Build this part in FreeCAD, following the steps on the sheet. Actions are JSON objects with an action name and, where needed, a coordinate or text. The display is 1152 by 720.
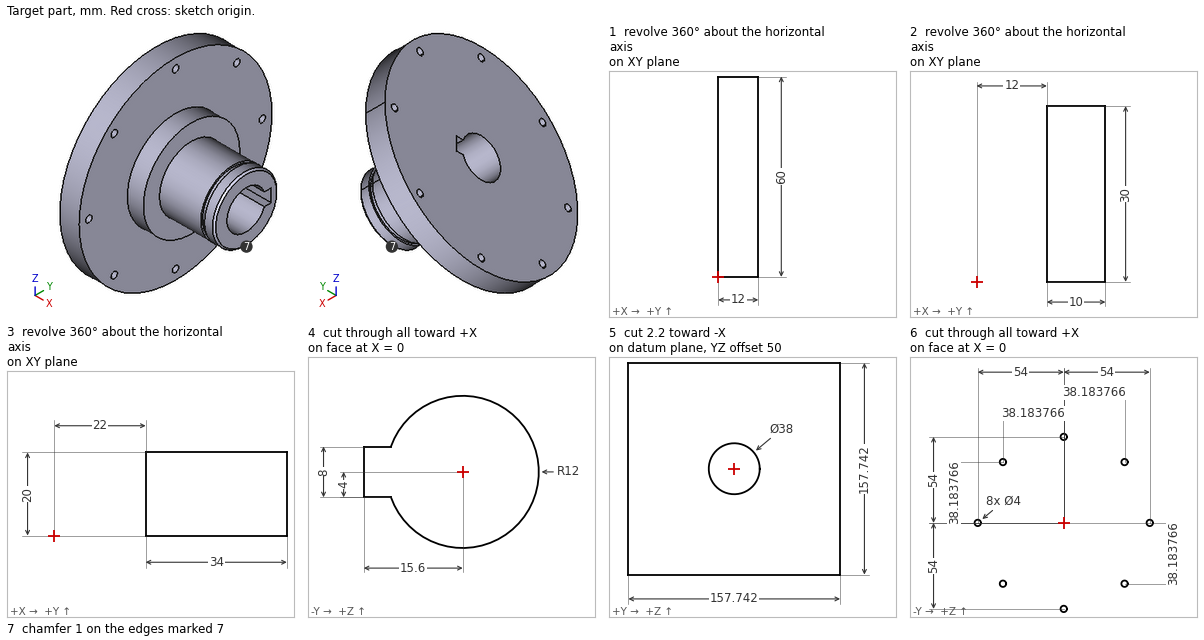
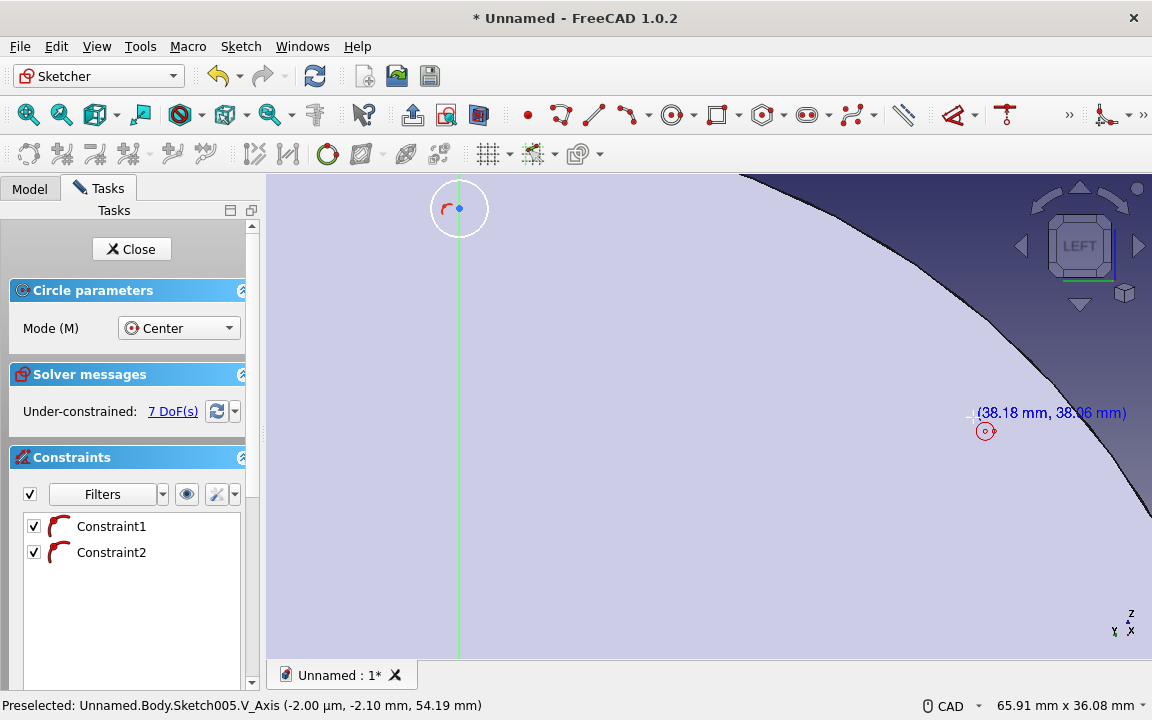
{"action": "scroll", "coordinate": [686, 287], "scroll_direction": "down", "scroll_amount": 8}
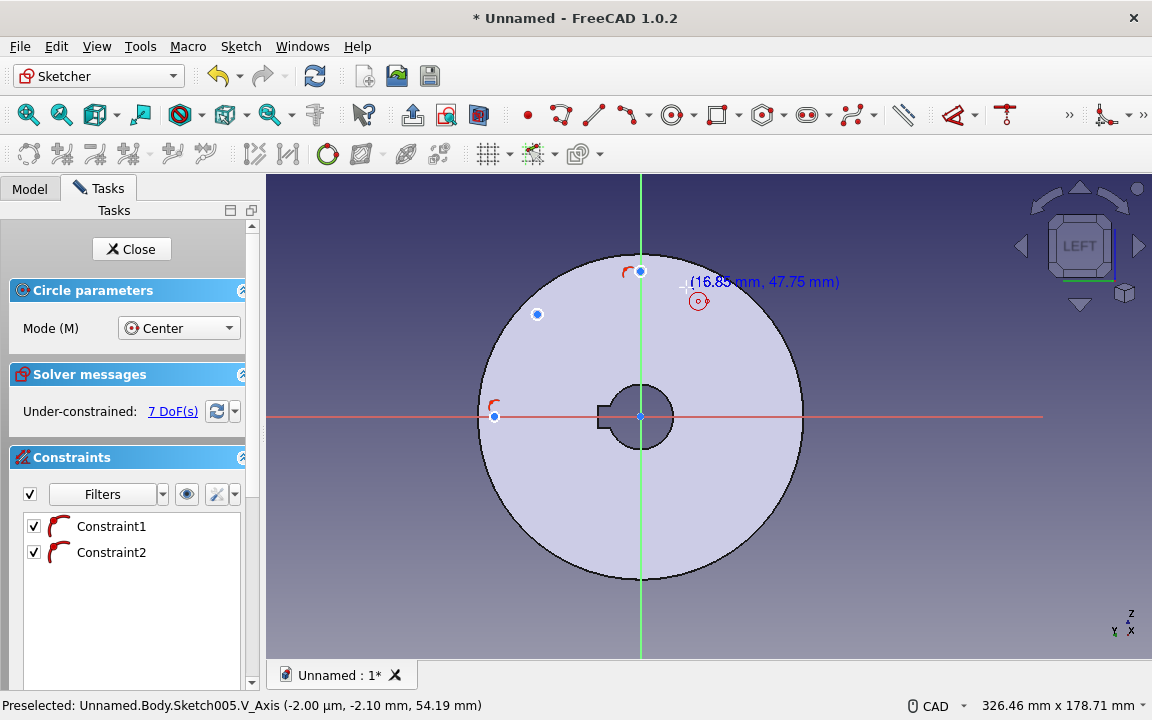
{"action": "left_click", "coordinate": [744, 313]}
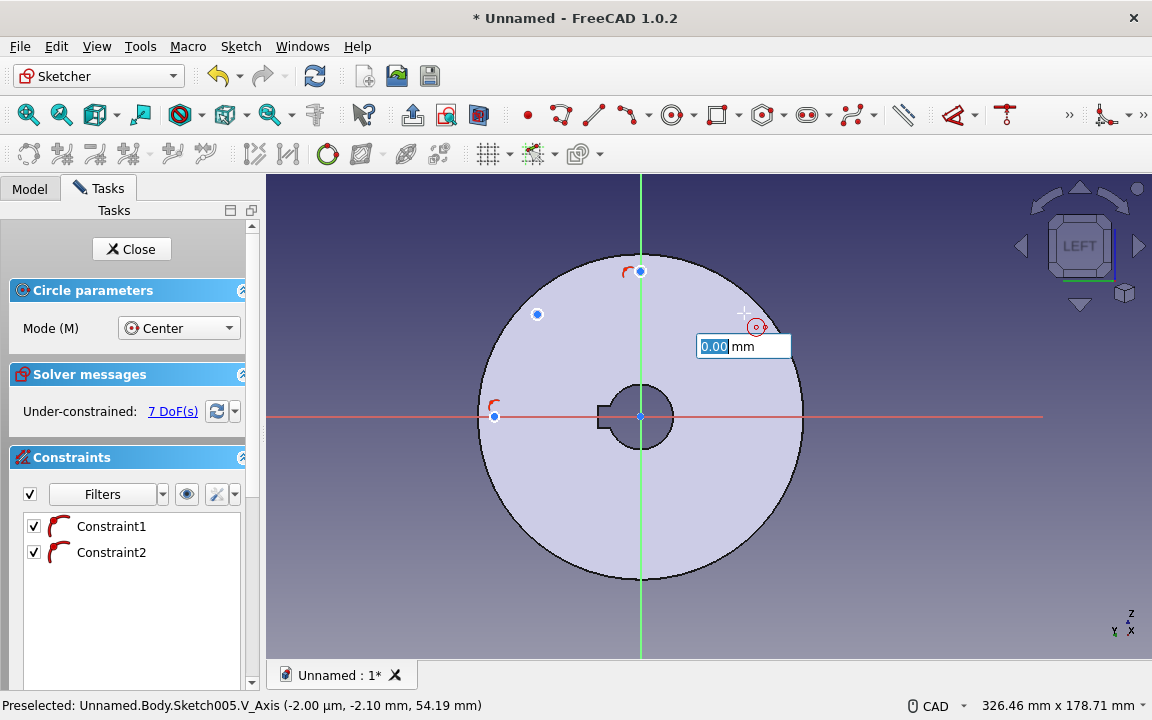
{"action": "scroll", "coordinate": [748, 310], "scroll_direction": "up", "scroll_amount": 6}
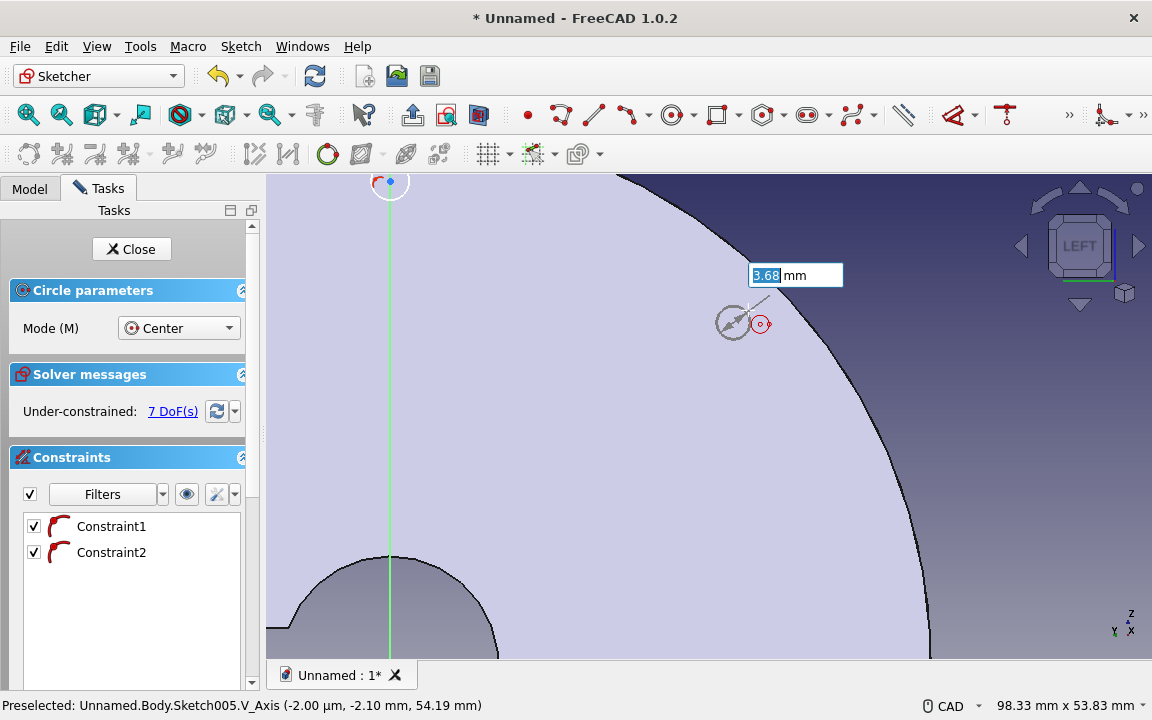
{"action": "left_click", "coordinate": [747, 308]}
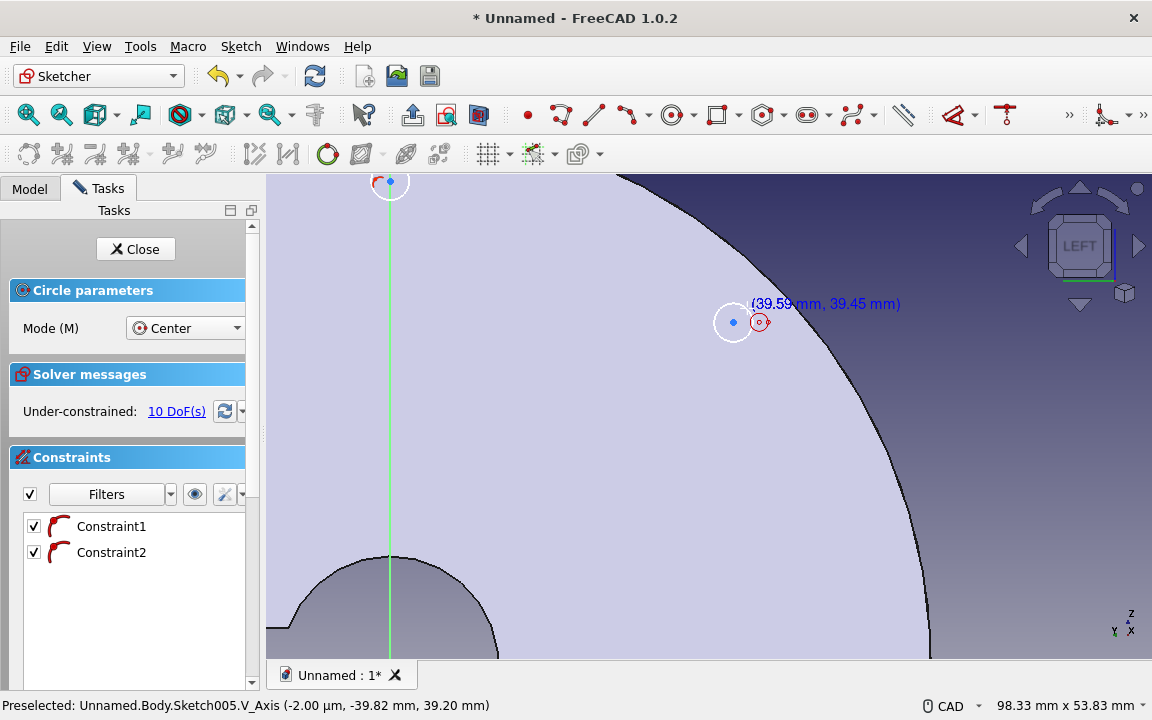
{"action": "scroll", "coordinate": [748, 310], "scroll_direction": "down", "scroll_amount": 6}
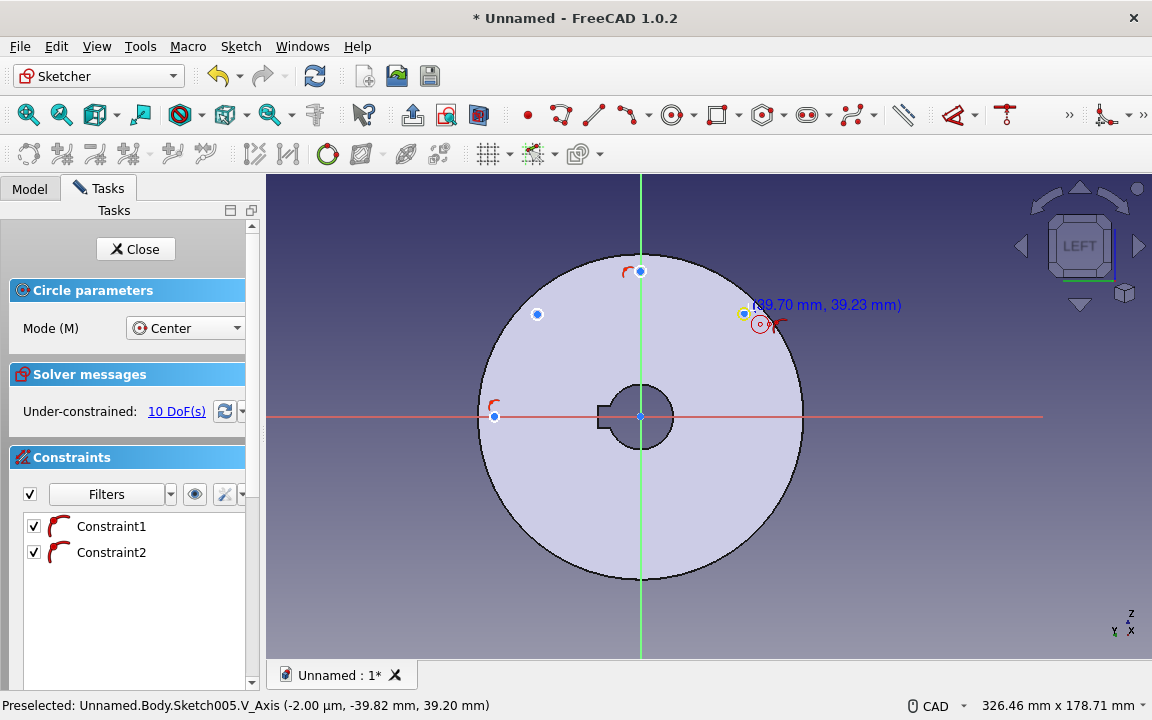
{"action": "scroll", "coordinate": [787, 417], "scroll_direction": "up", "scroll_amount": 8}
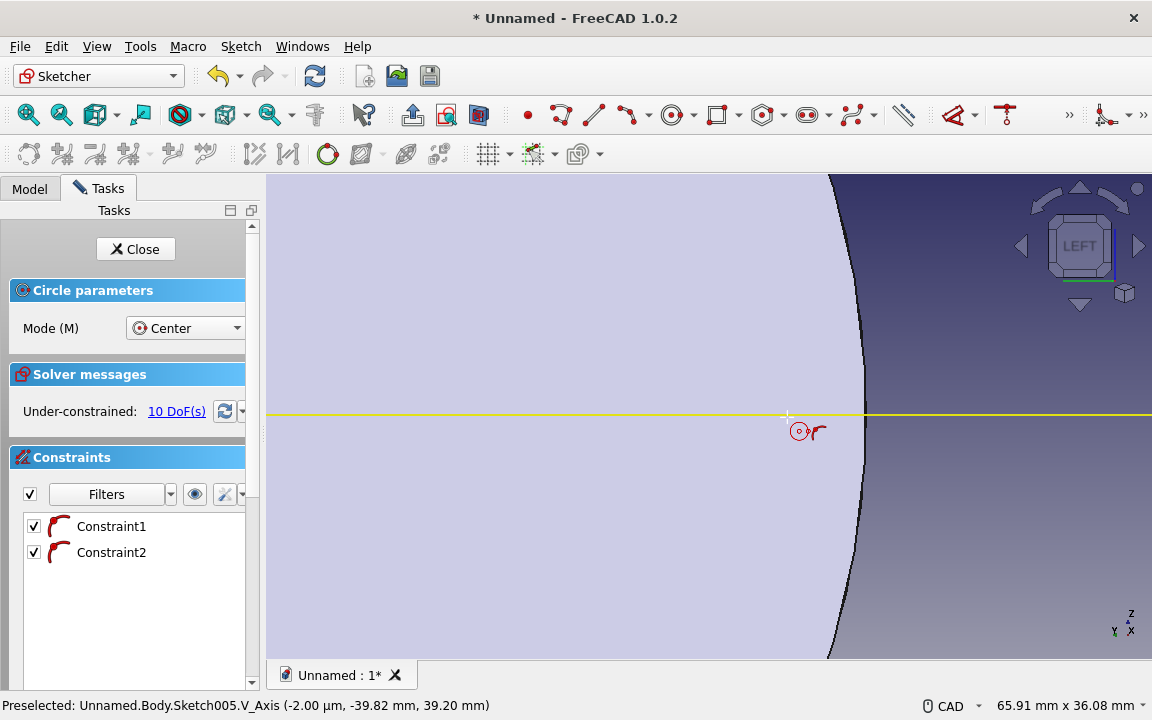
{"action": "scroll", "coordinate": [787, 417], "scroll_direction": "down", "scroll_amount": 8}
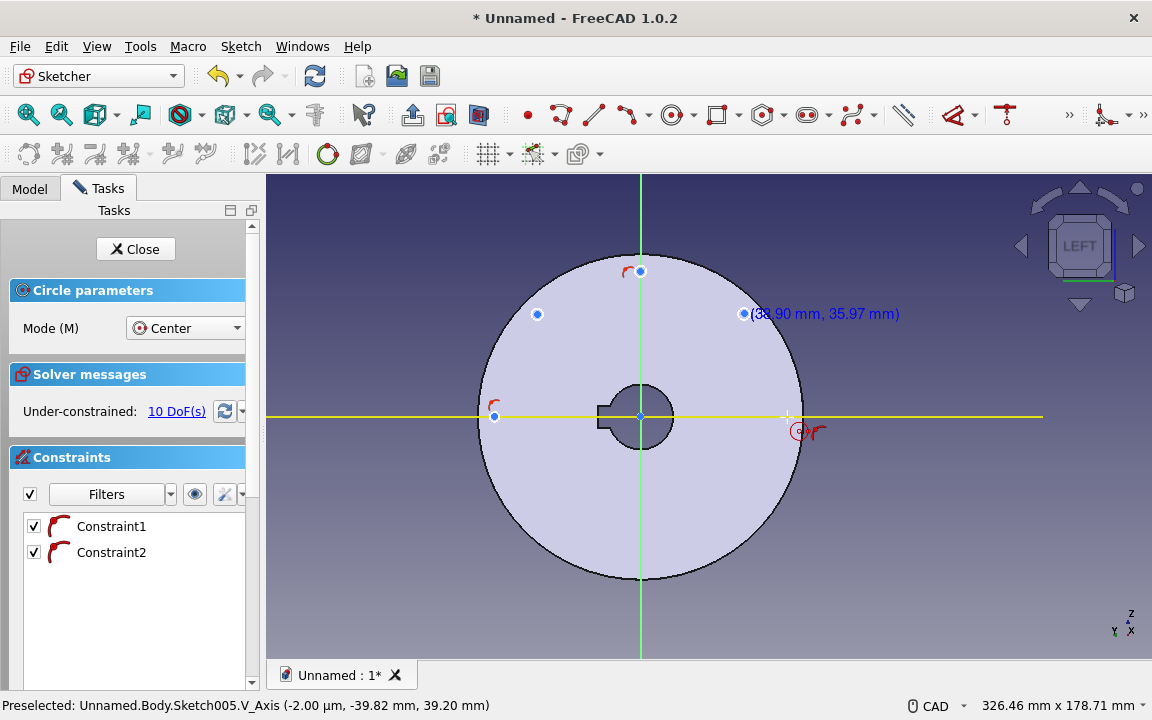
{"action": "left_click", "coordinate": [787, 417]}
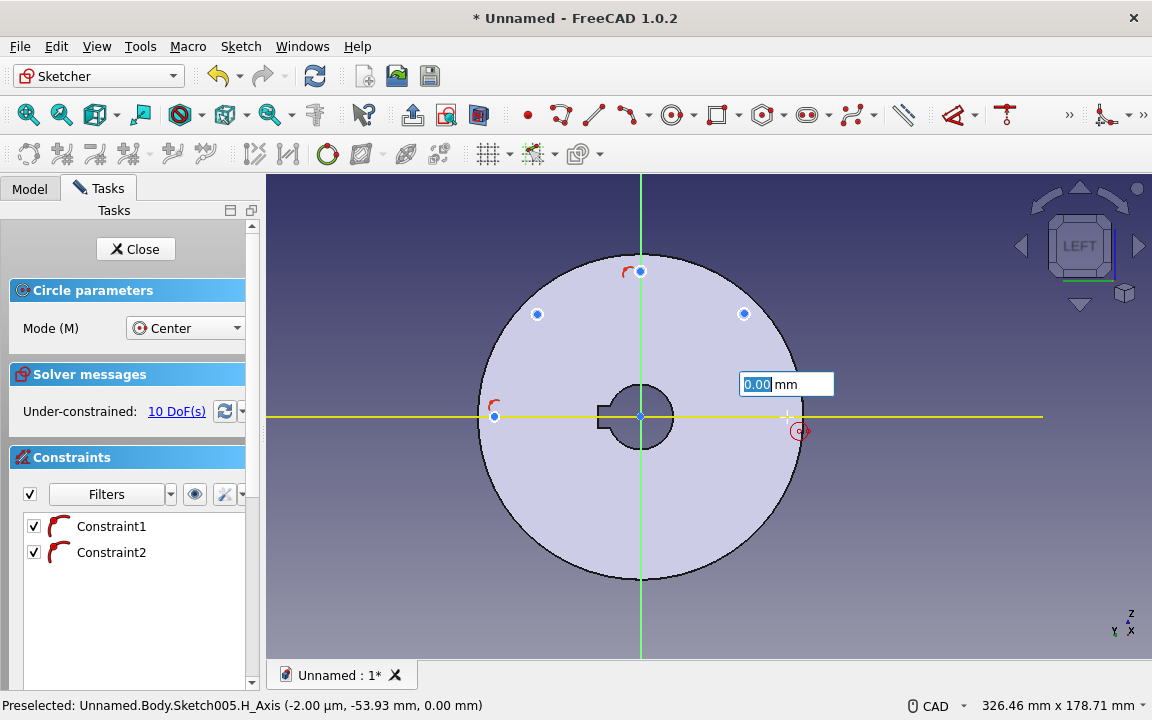
{"action": "scroll", "coordinate": [785, 422], "scroll_direction": "up", "scroll_amount": 6}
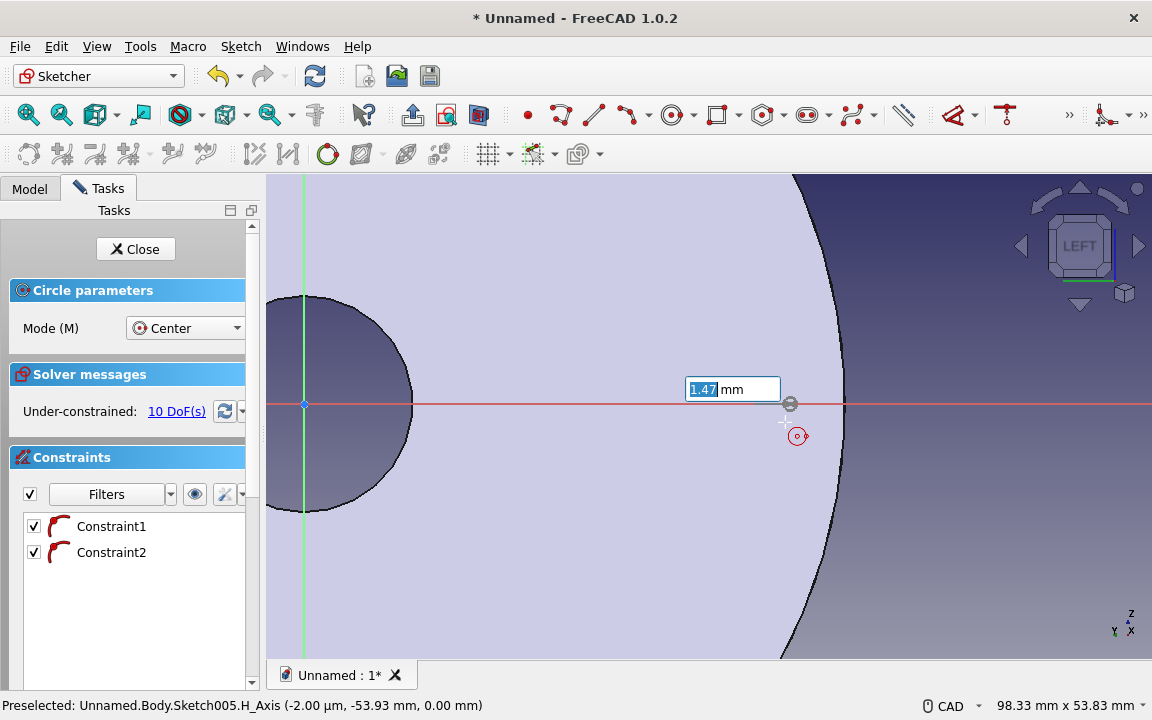
{"action": "left_click", "coordinate": [785, 421]}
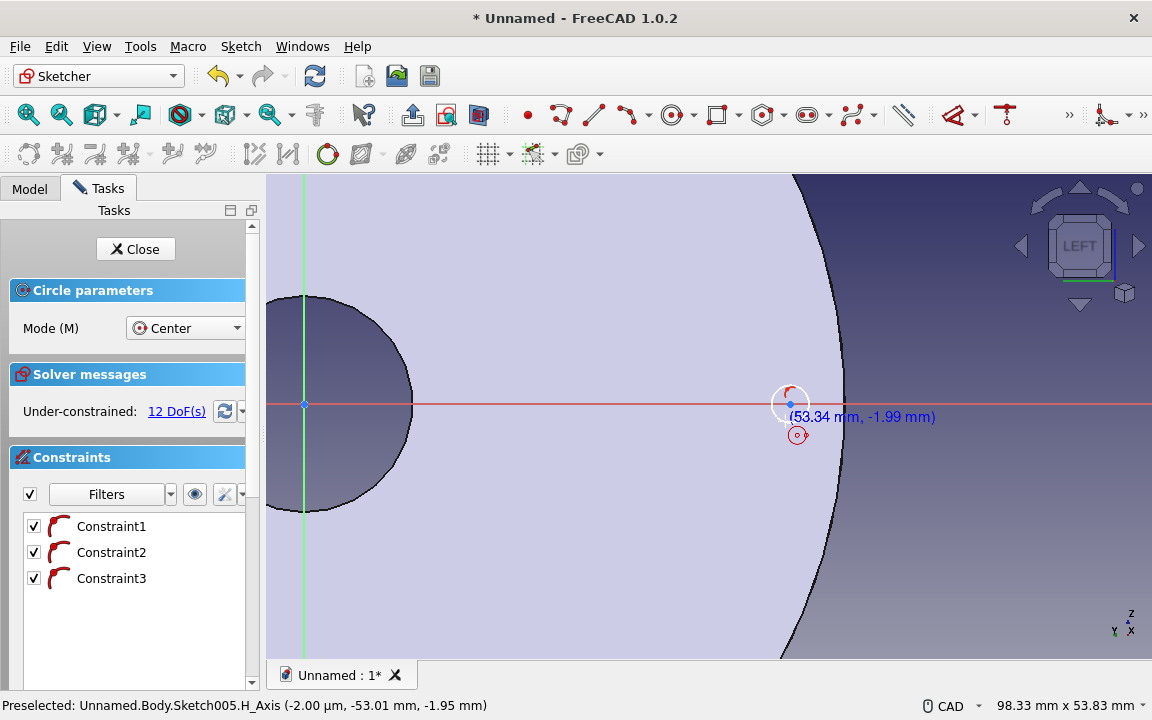
{"action": "scroll", "coordinate": [785, 422], "scroll_direction": "down", "scroll_amount": 6}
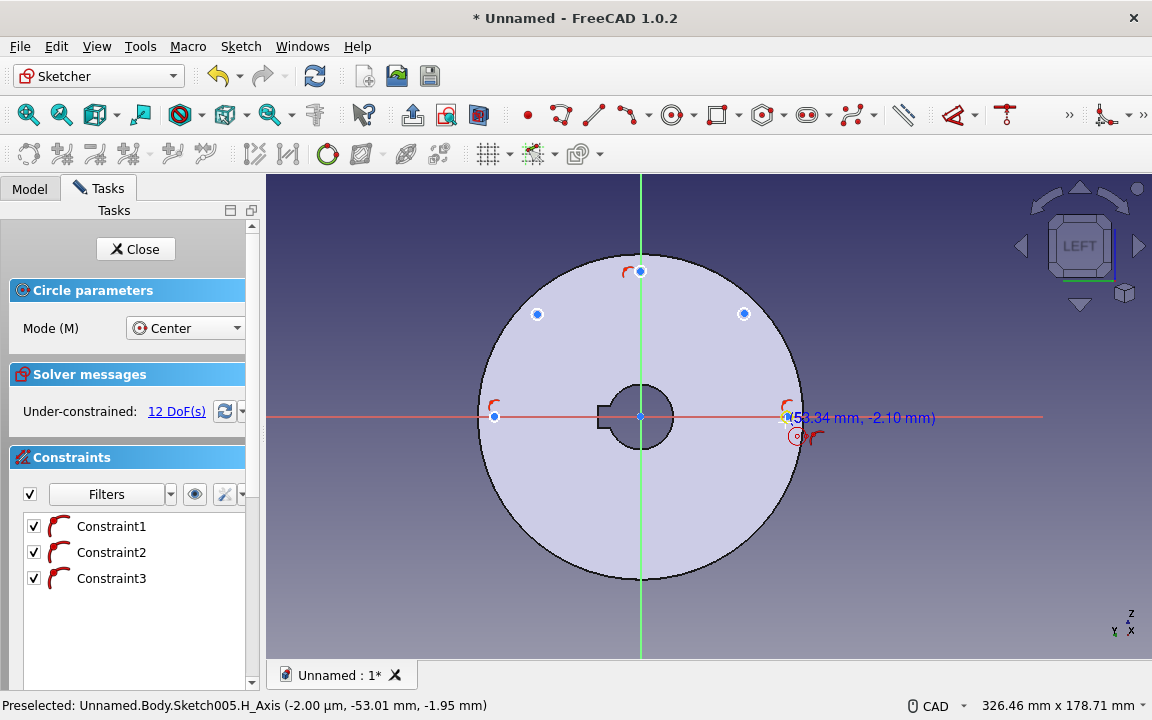
{"action": "scroll", "coordinate": [744, 521], "scroll_direction": "up", "scroll_amount": 8}